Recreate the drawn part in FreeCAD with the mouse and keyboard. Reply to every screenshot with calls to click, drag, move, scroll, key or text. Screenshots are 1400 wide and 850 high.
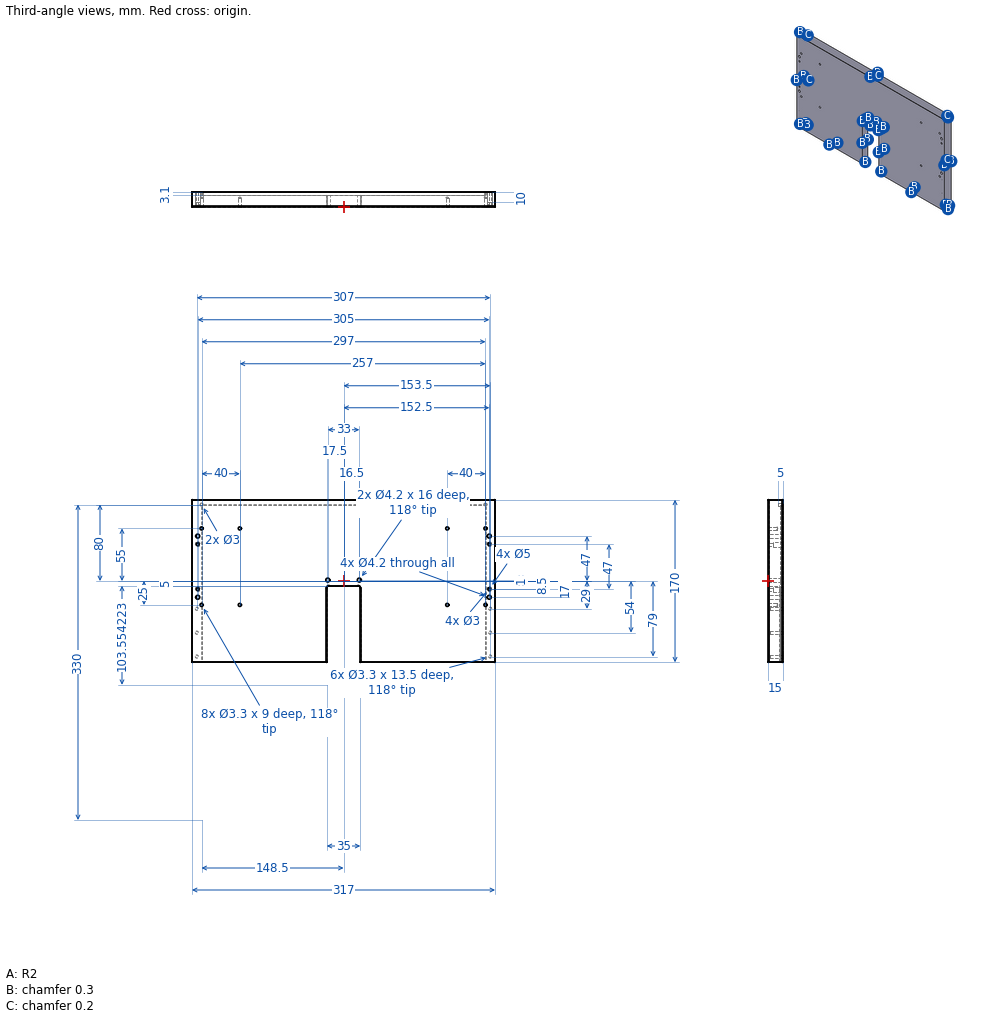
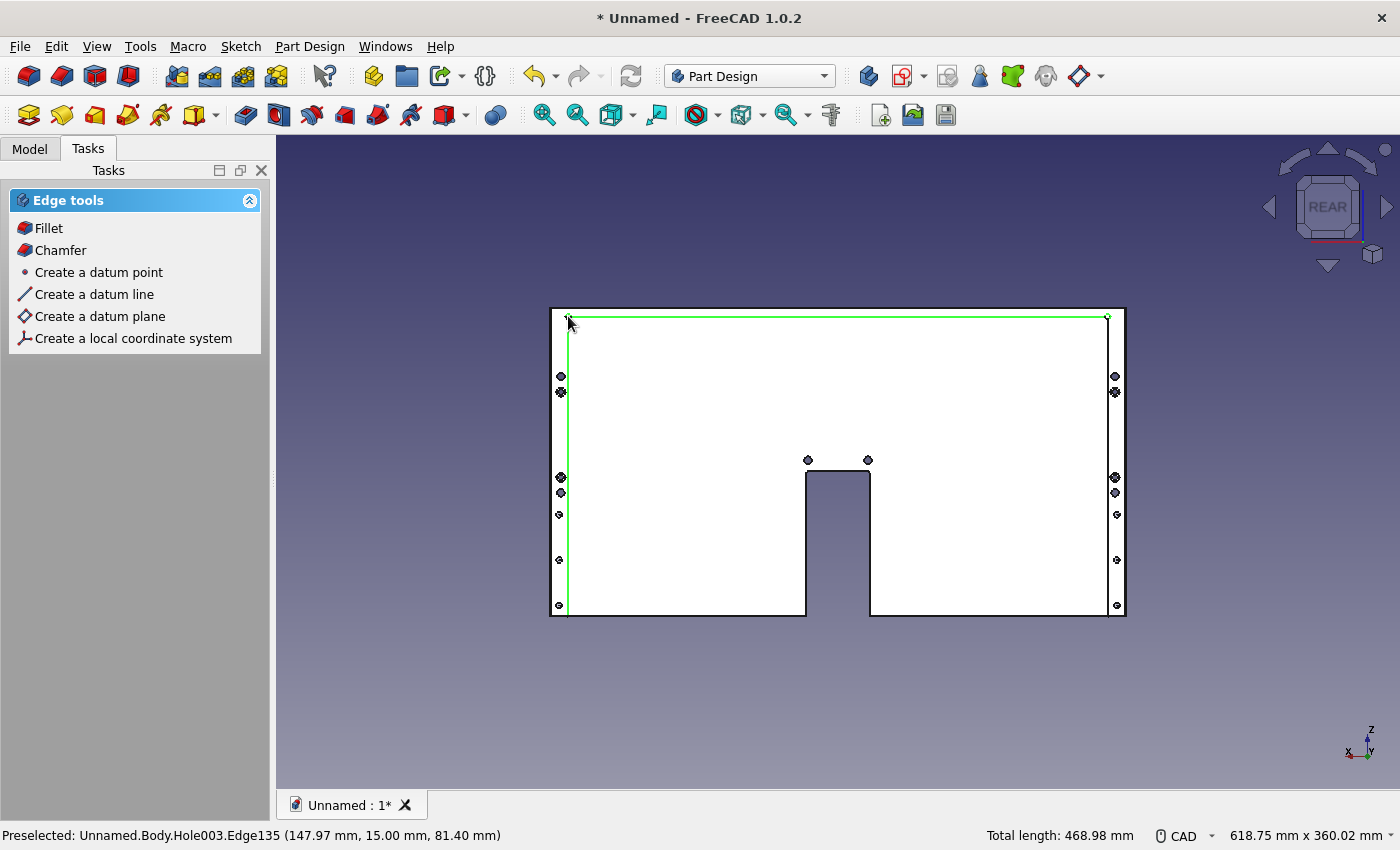
click(1108, 467, ctrl)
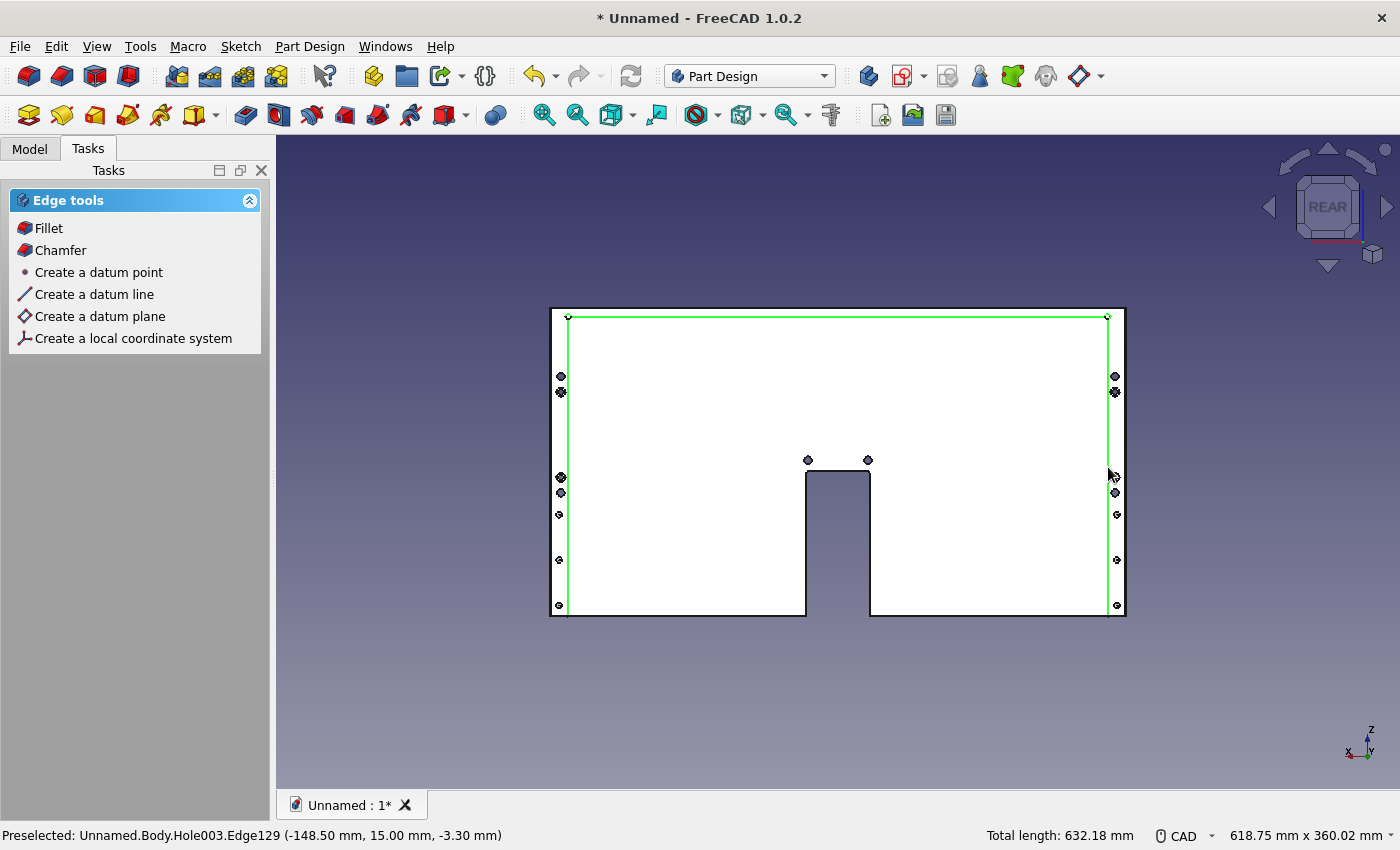
click(62, 76)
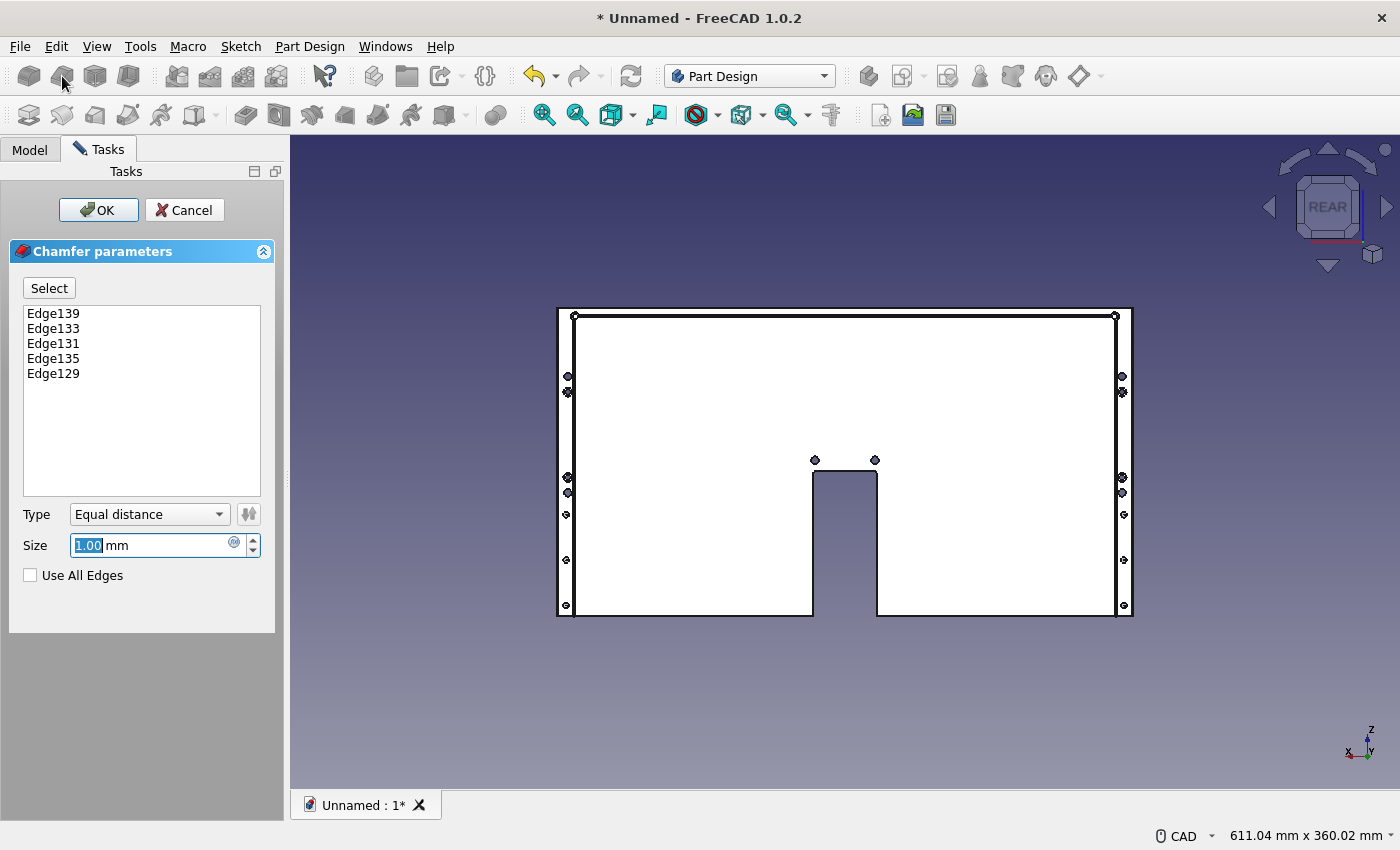
text(0.2)
key(Tab)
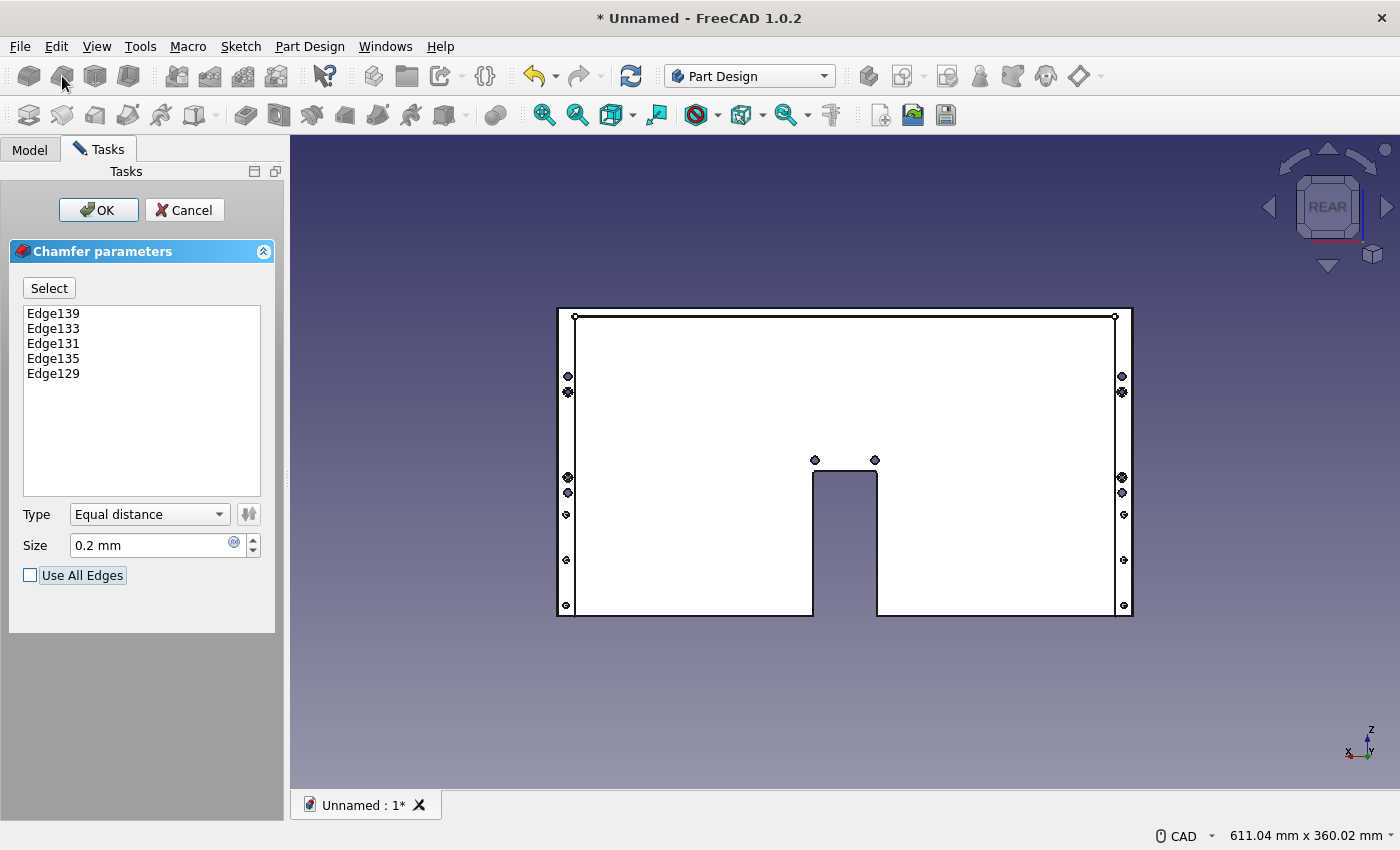
click(99, 210)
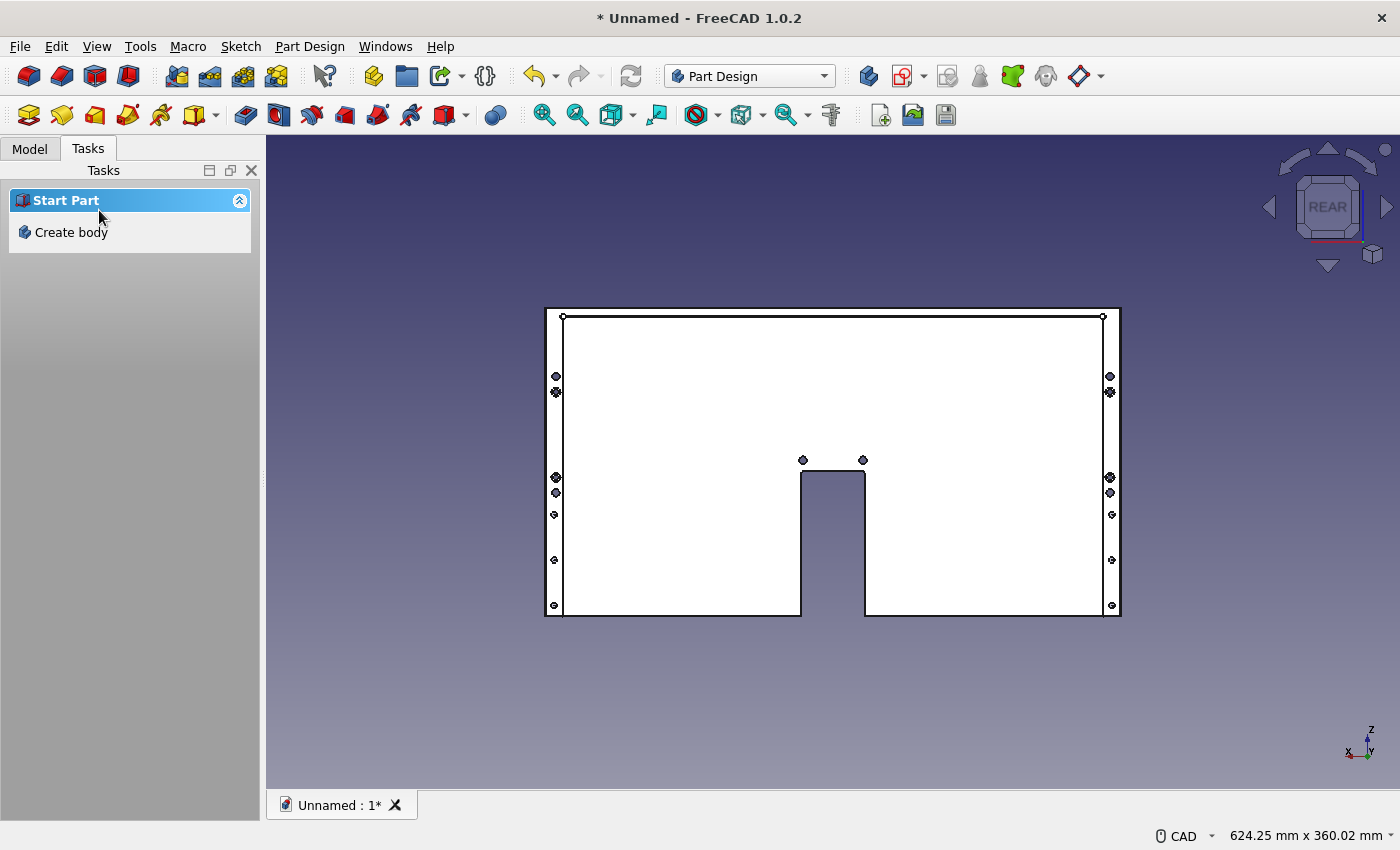
key(0)